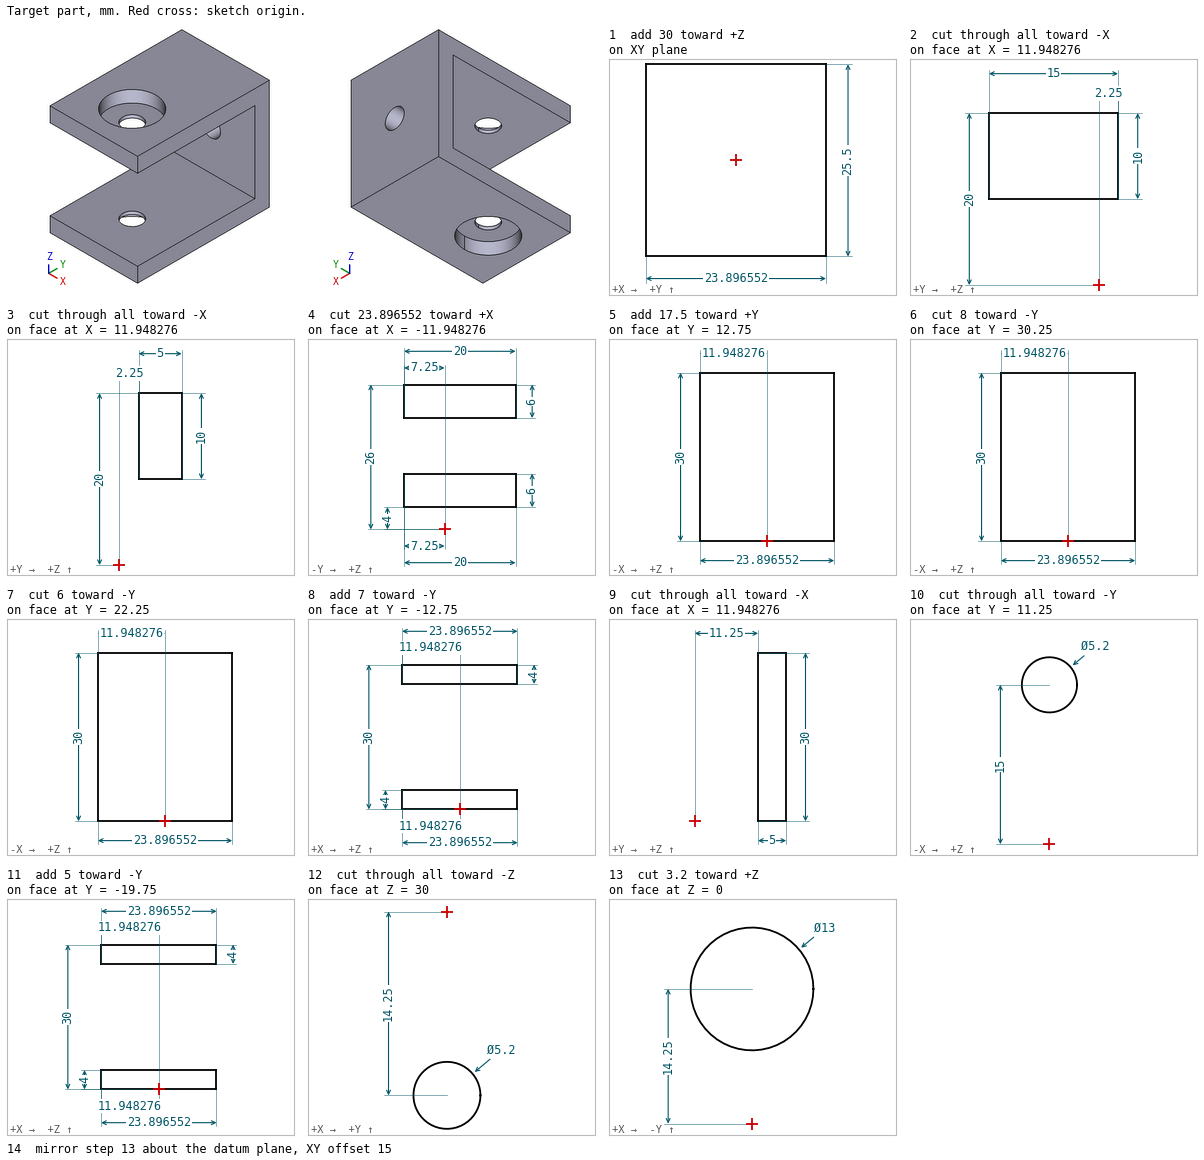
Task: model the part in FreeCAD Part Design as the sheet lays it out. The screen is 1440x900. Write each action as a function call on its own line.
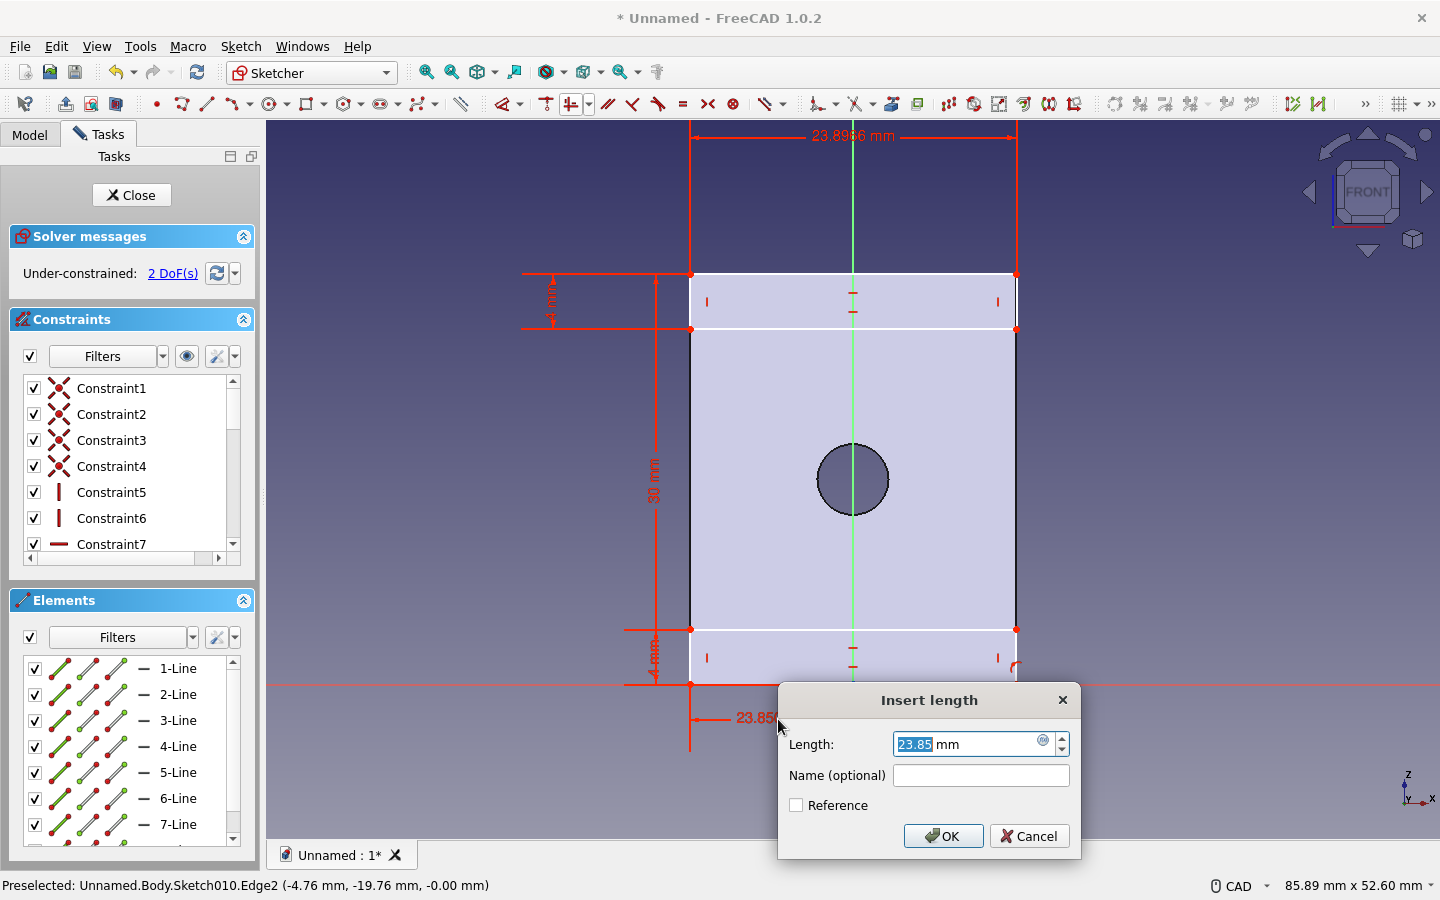
text(23.896552)
key(Return)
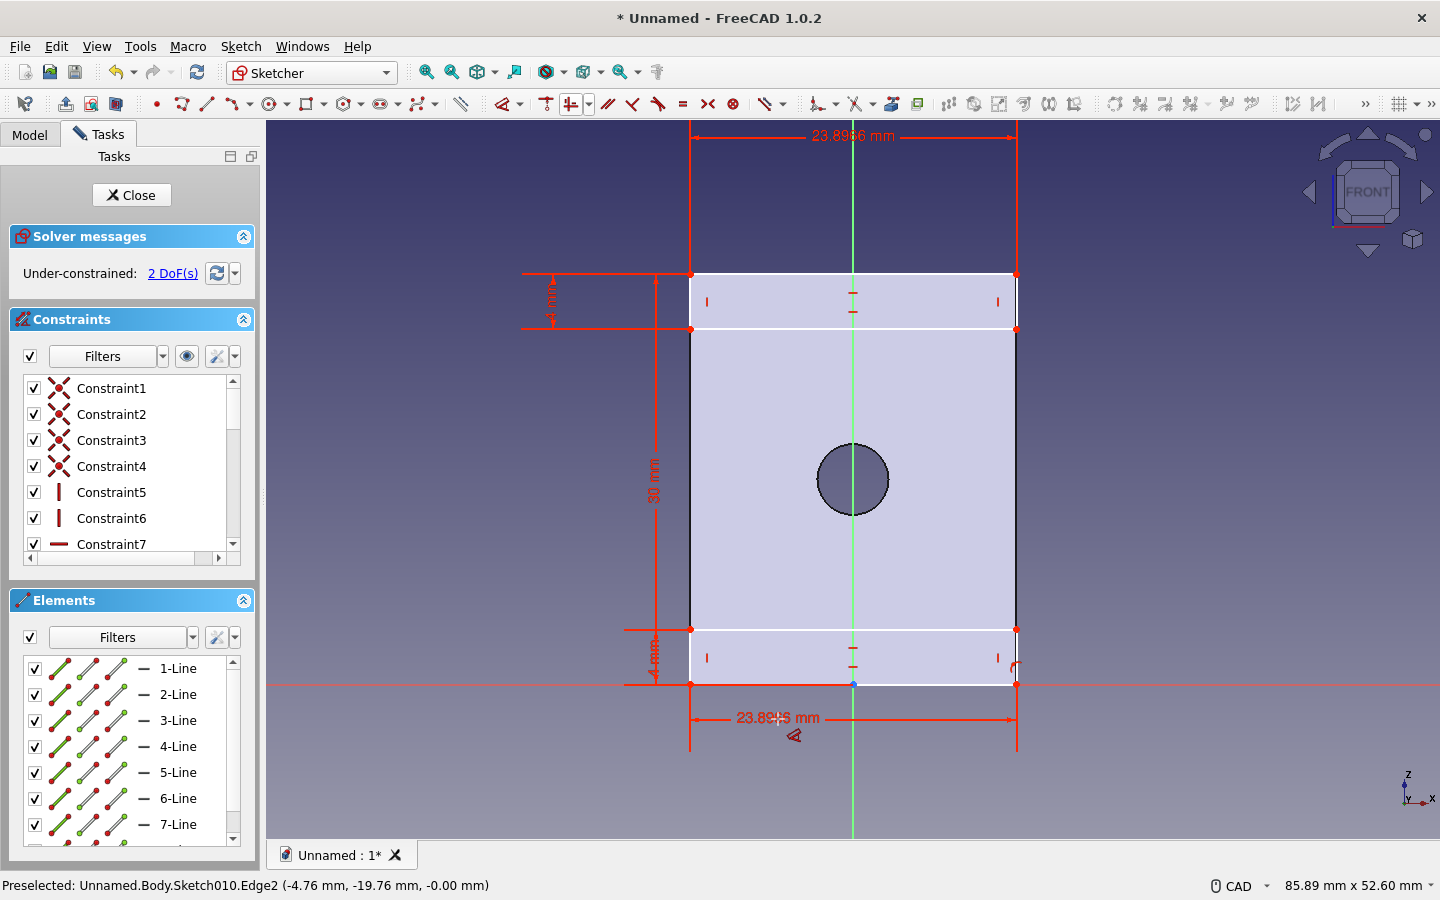
click(690, 630)
click(771, 596)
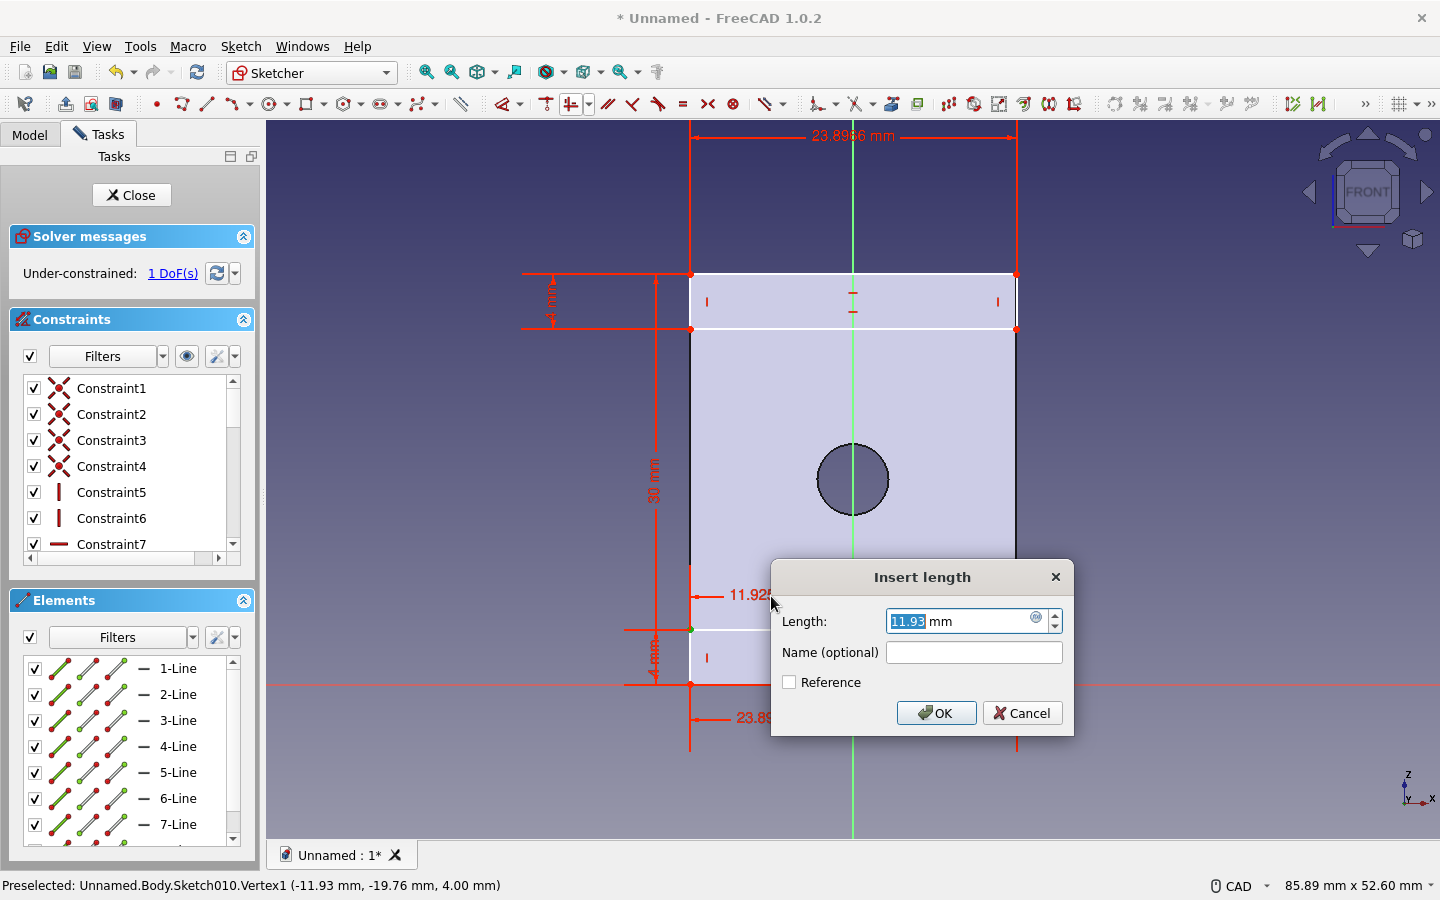
text(11.948276)
key(Return)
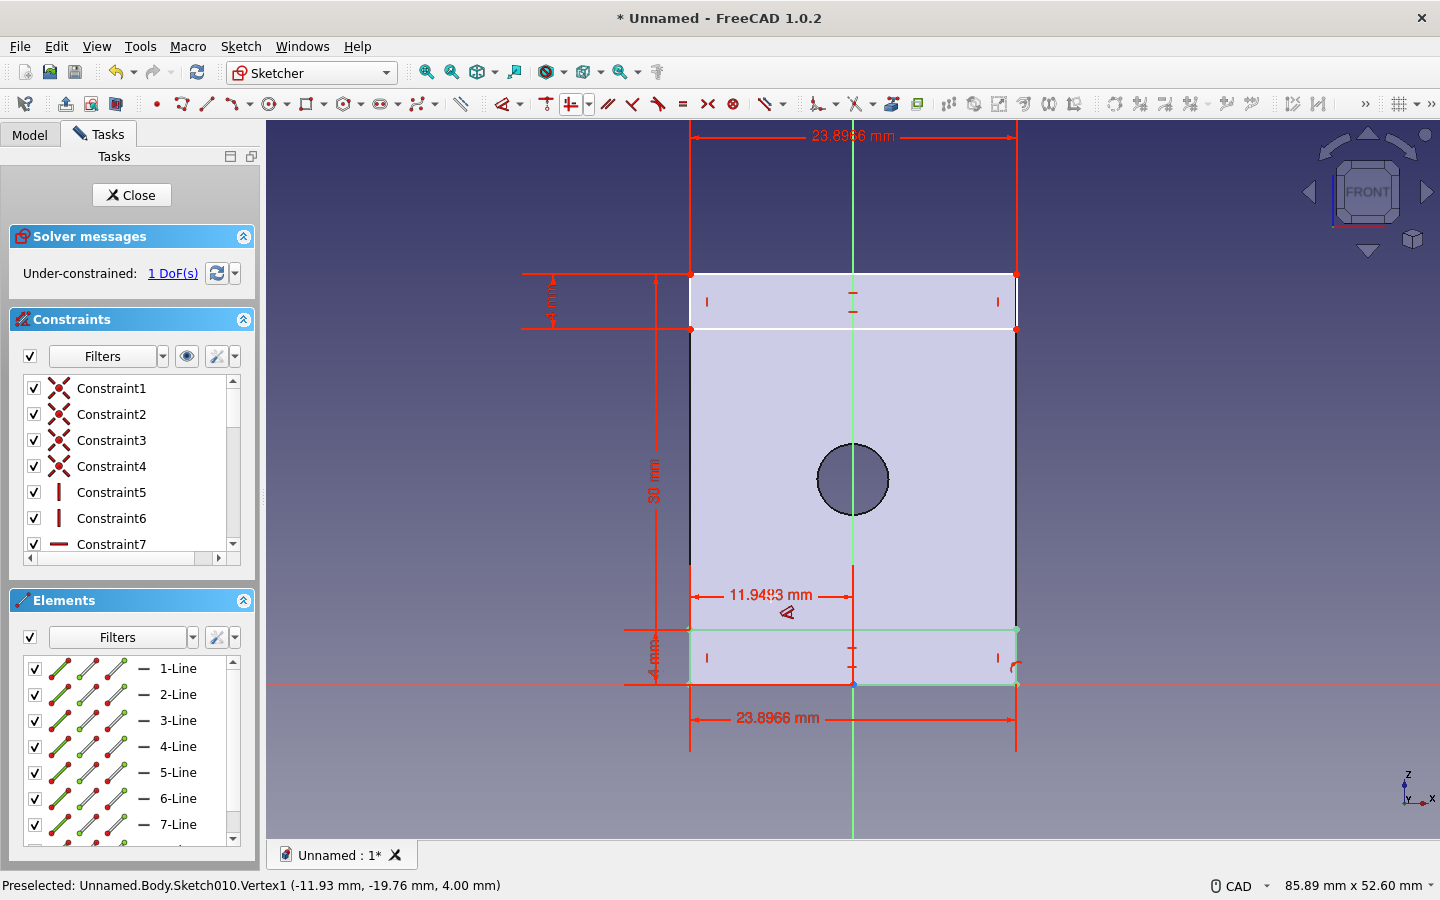
click(690, 274)
click(771, 240)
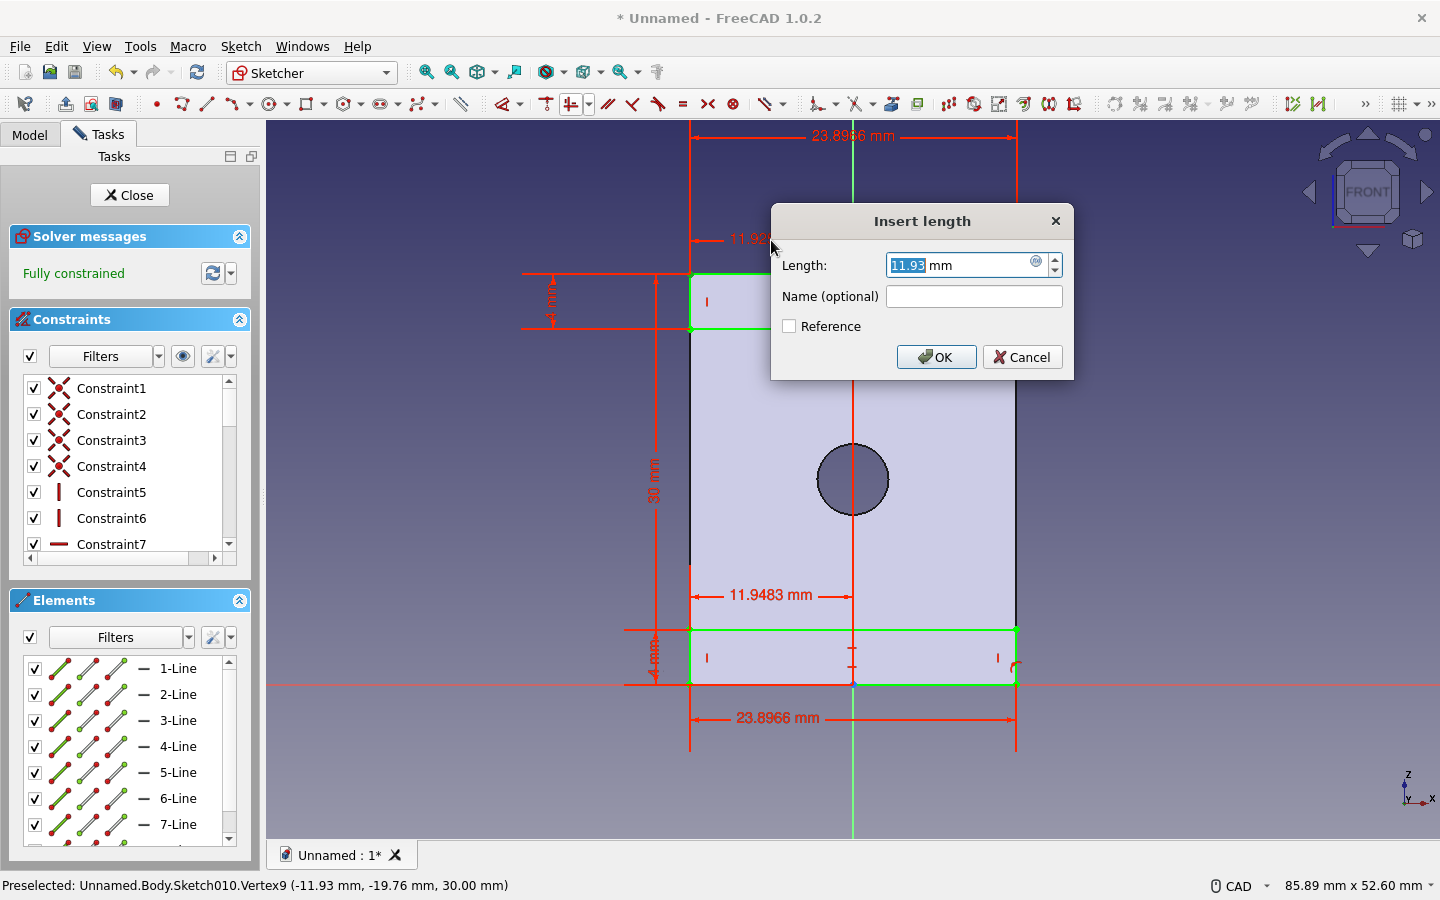
text(11.948276)
key(Return)
key(Escape)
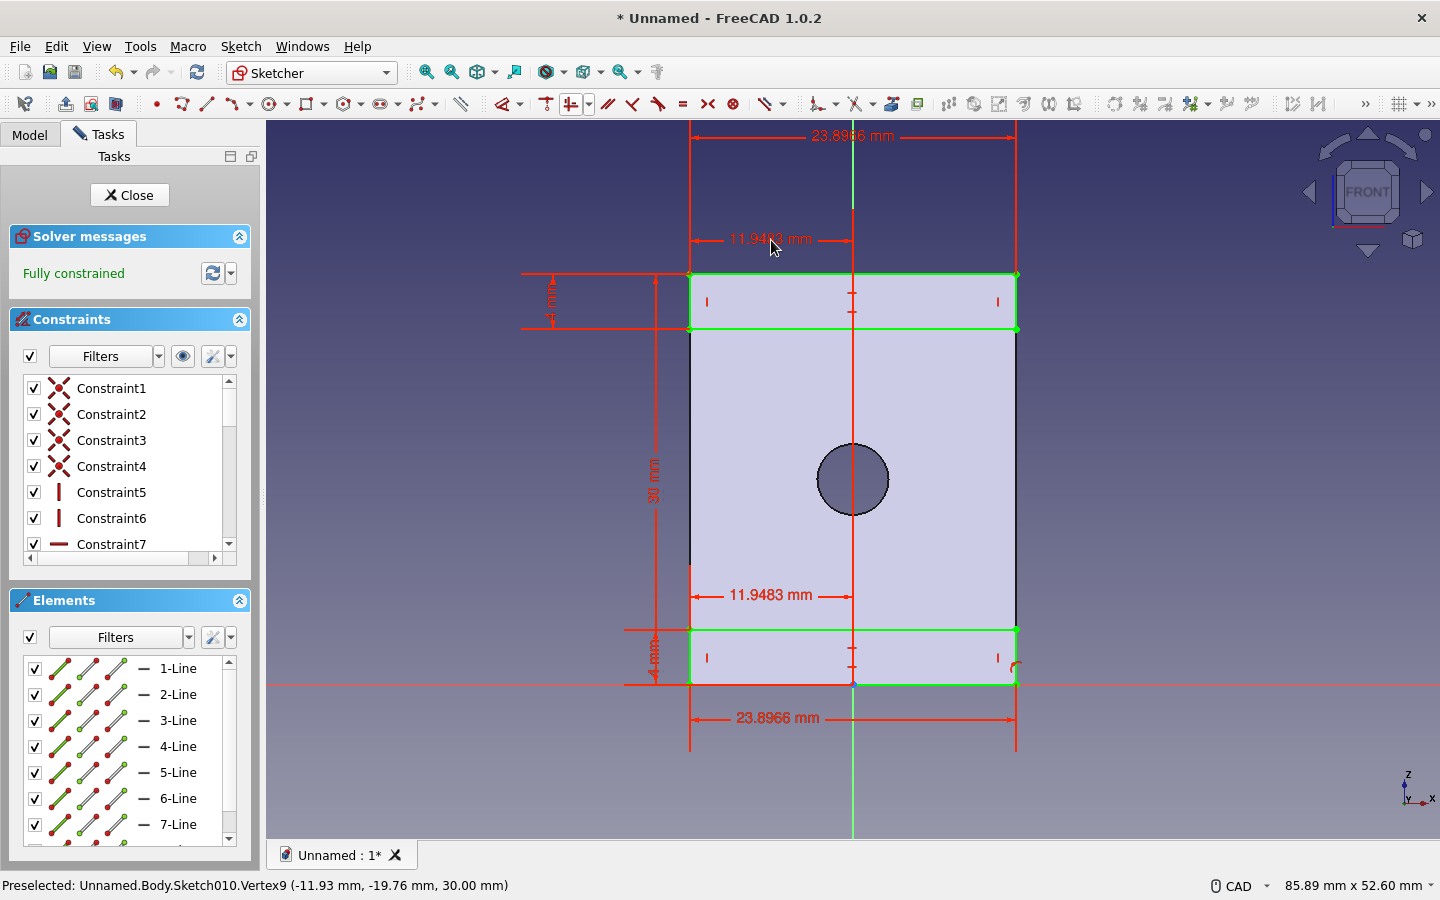
click(130, 195)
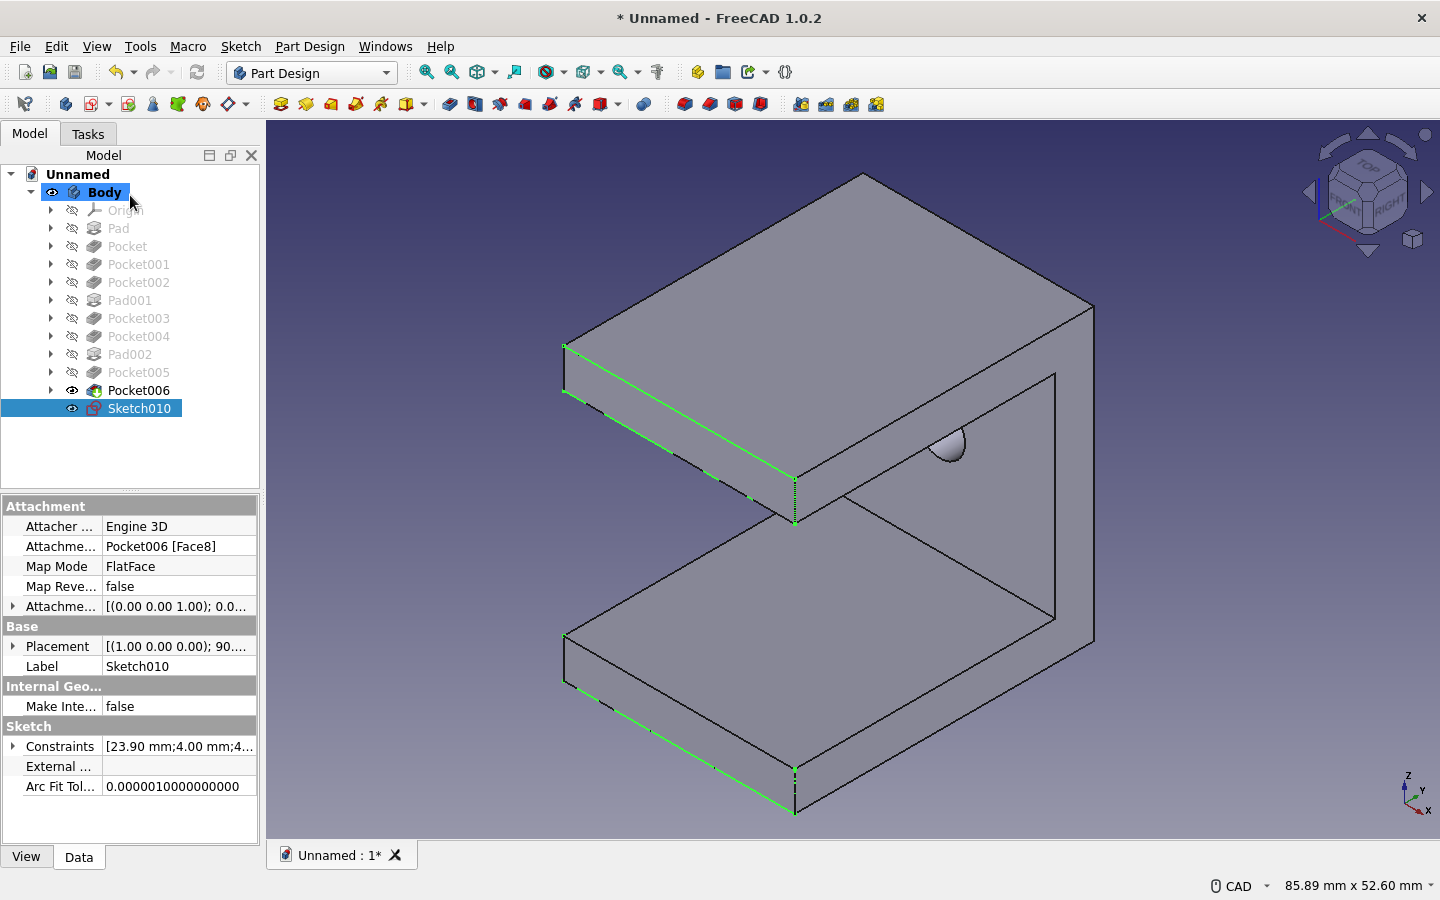
click(281, 104)